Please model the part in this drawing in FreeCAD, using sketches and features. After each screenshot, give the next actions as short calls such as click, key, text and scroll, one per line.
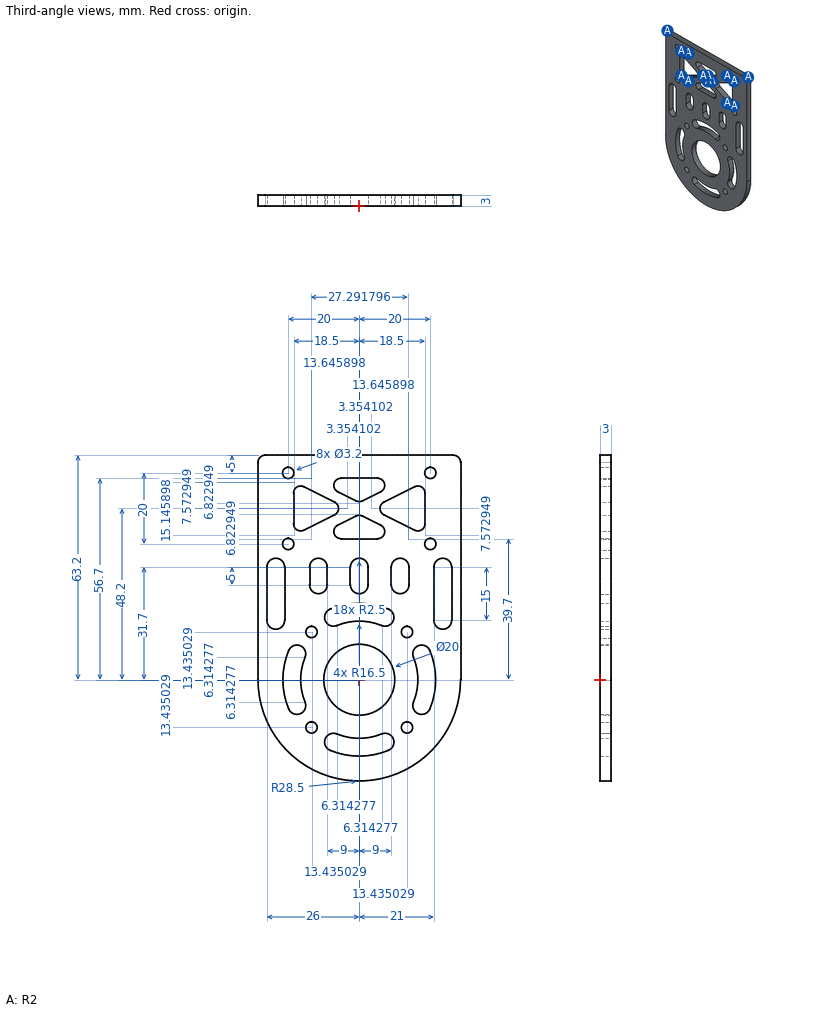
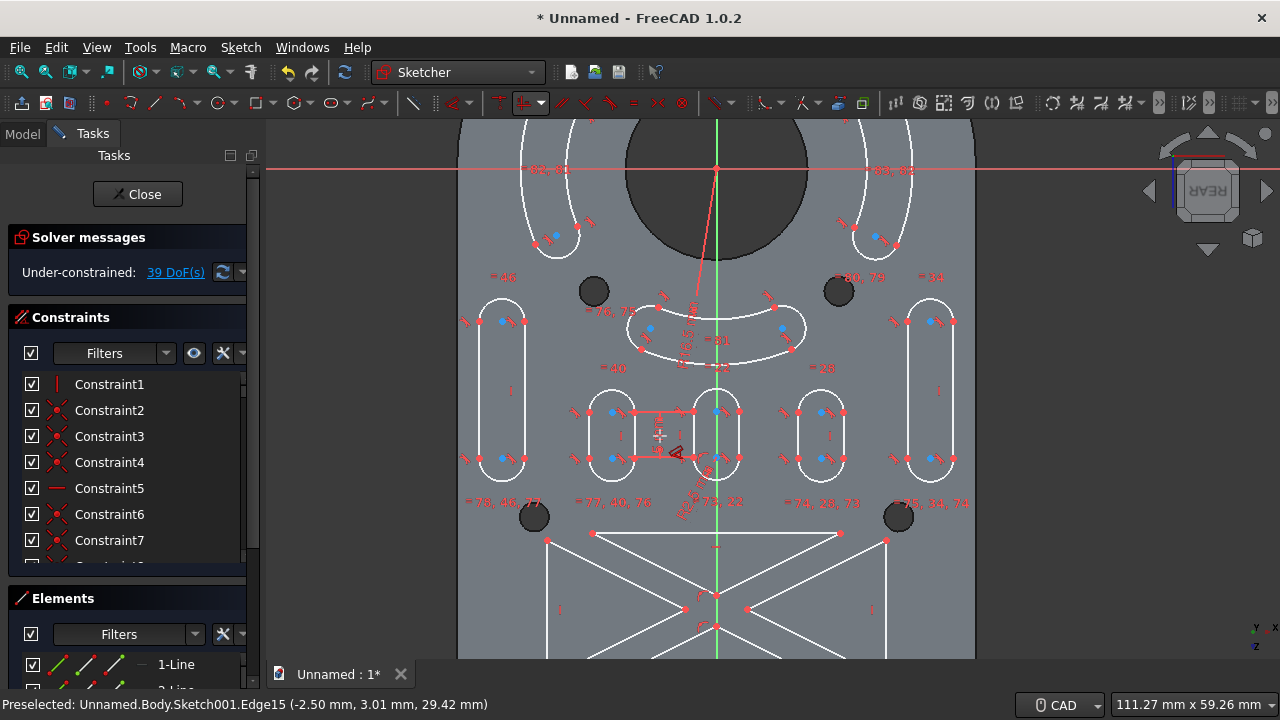
click(798, 445)
click(764, 436)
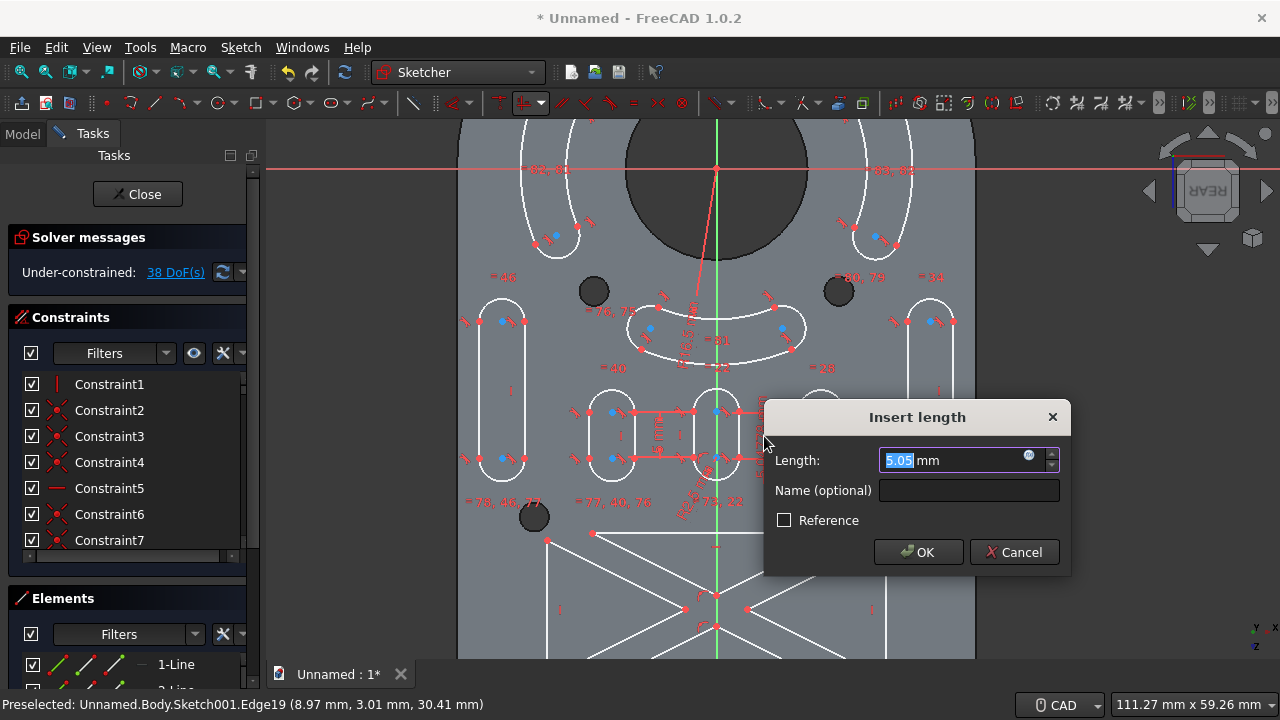
text(5)
key(Return)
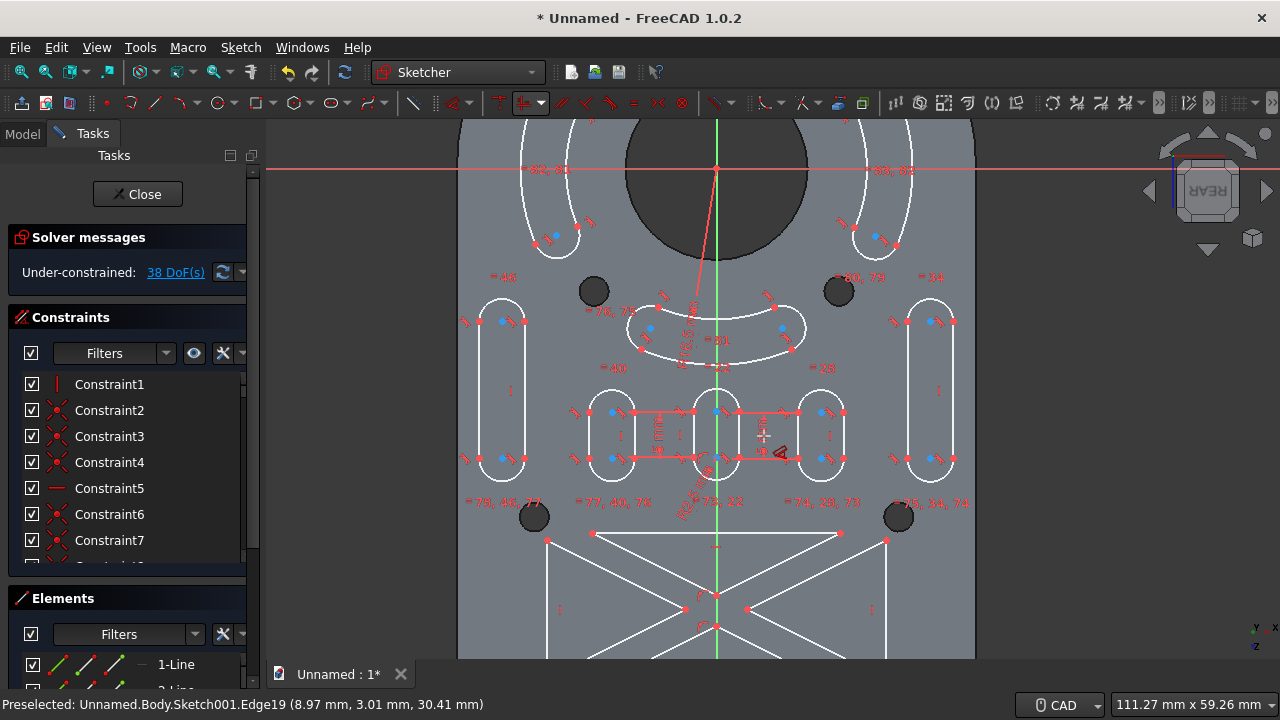
click(589, 445)
click(555, 436)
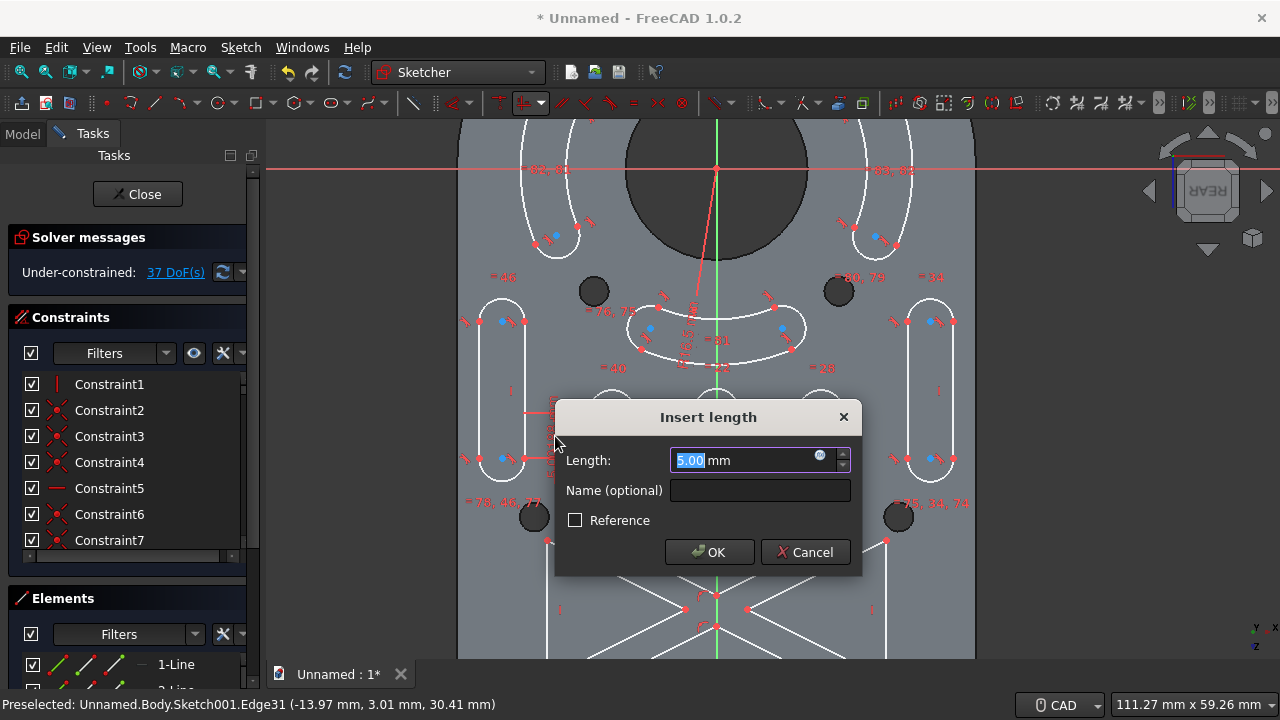
text(5)
key(Return)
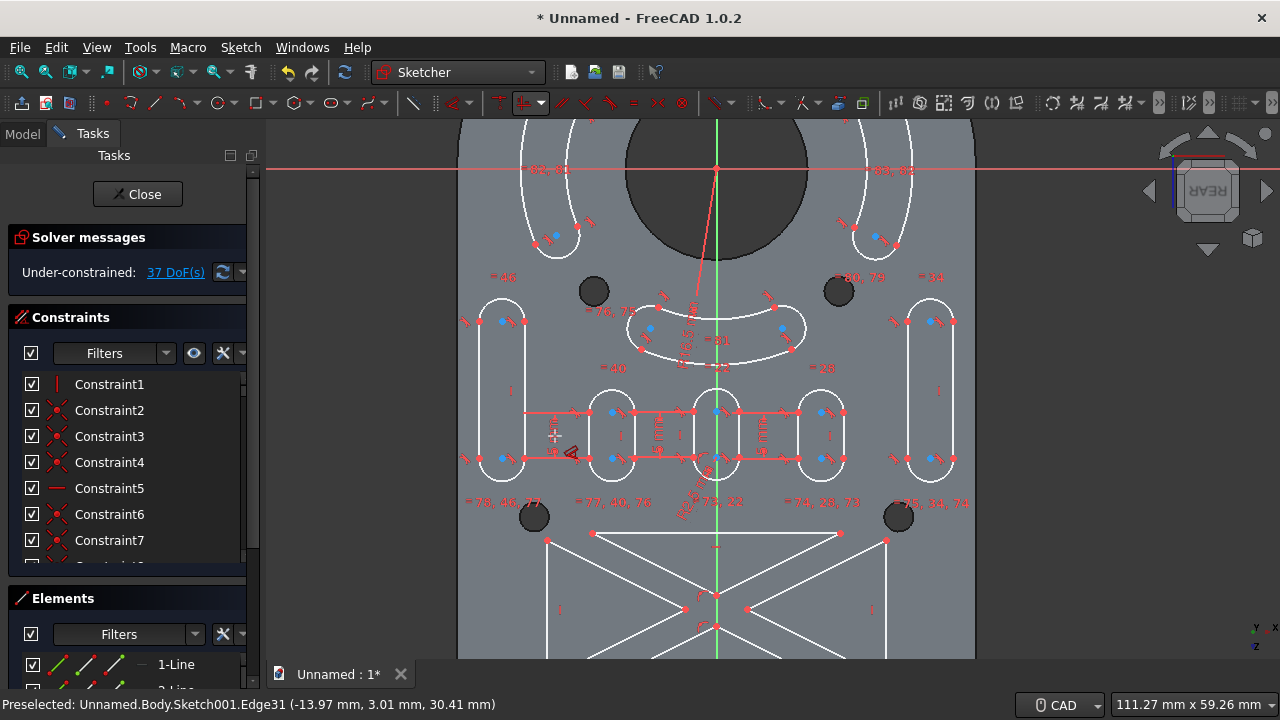
click(908, 418)
click(874, 390)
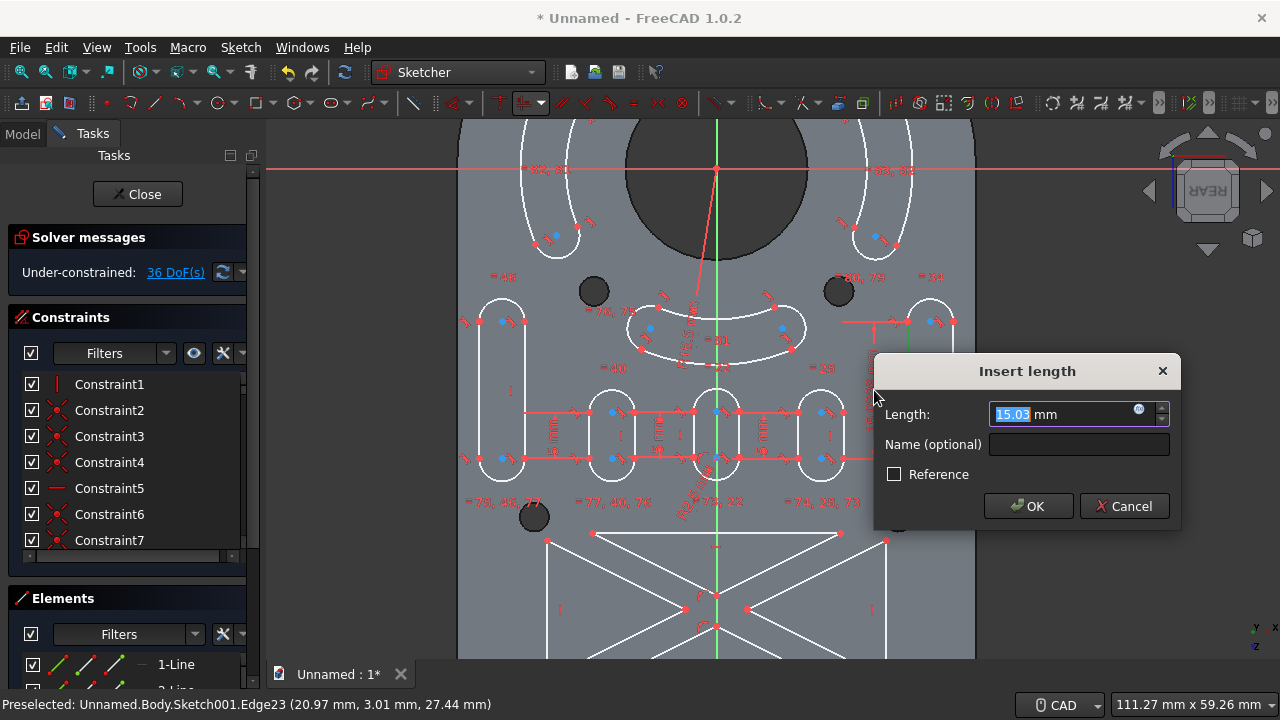
text(15)
key(Return)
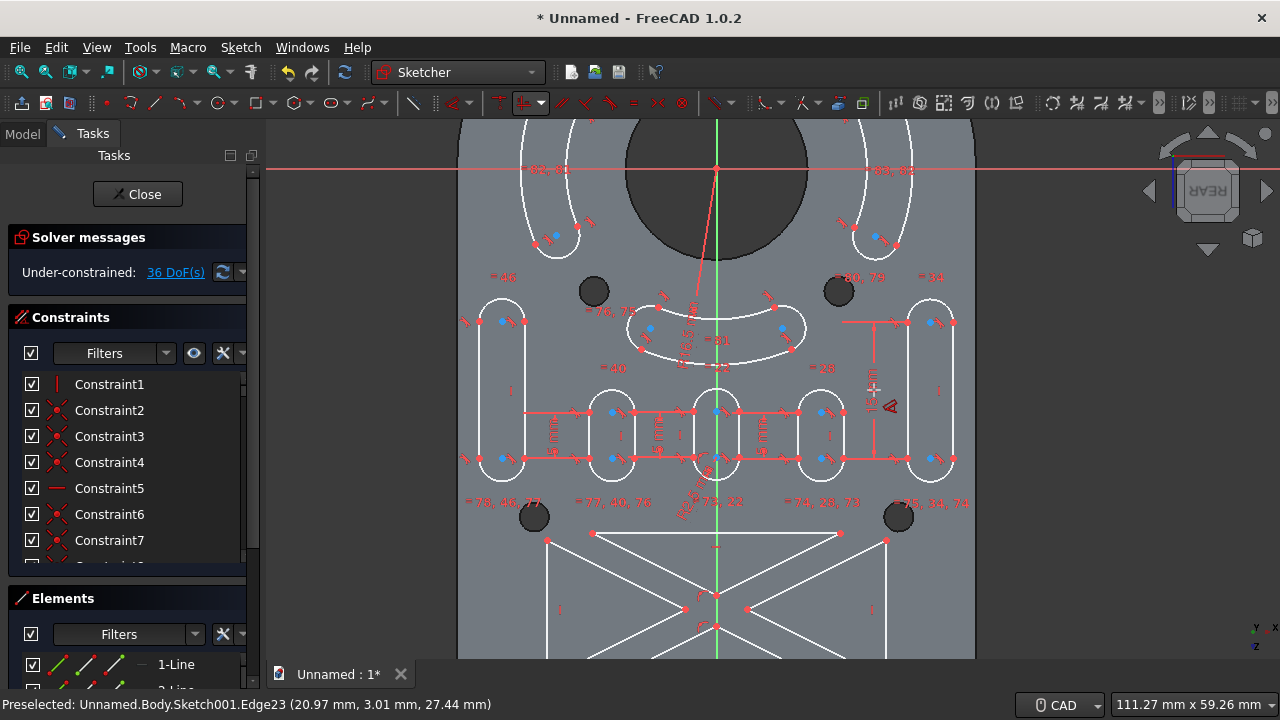
click(479, 417)
click(445, 390)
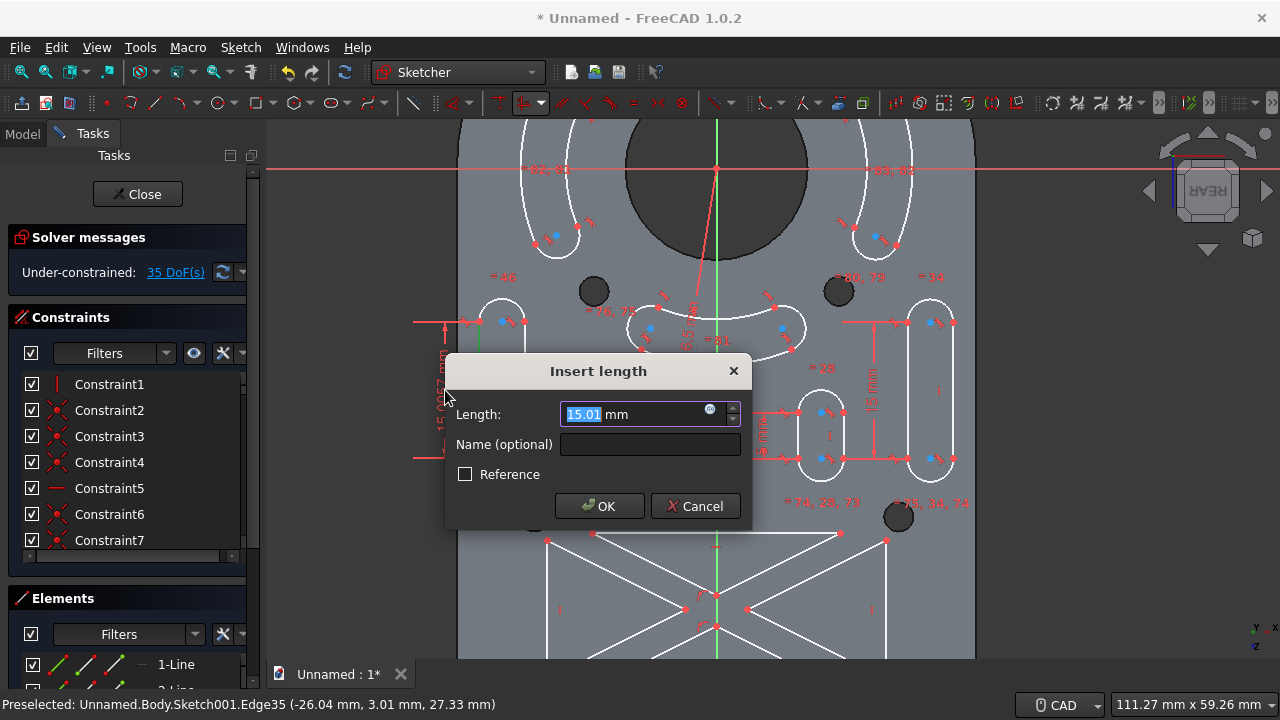
text(15)
key(Return)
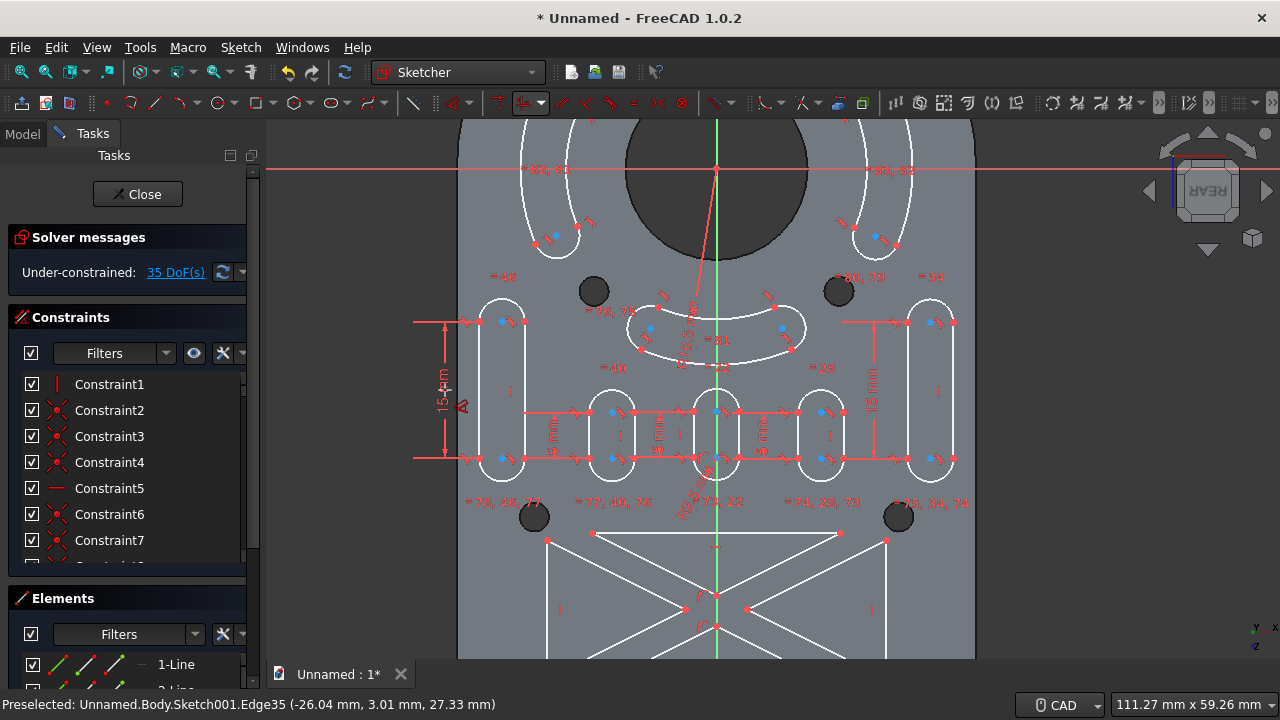
click(798, 459)
click(776, 493)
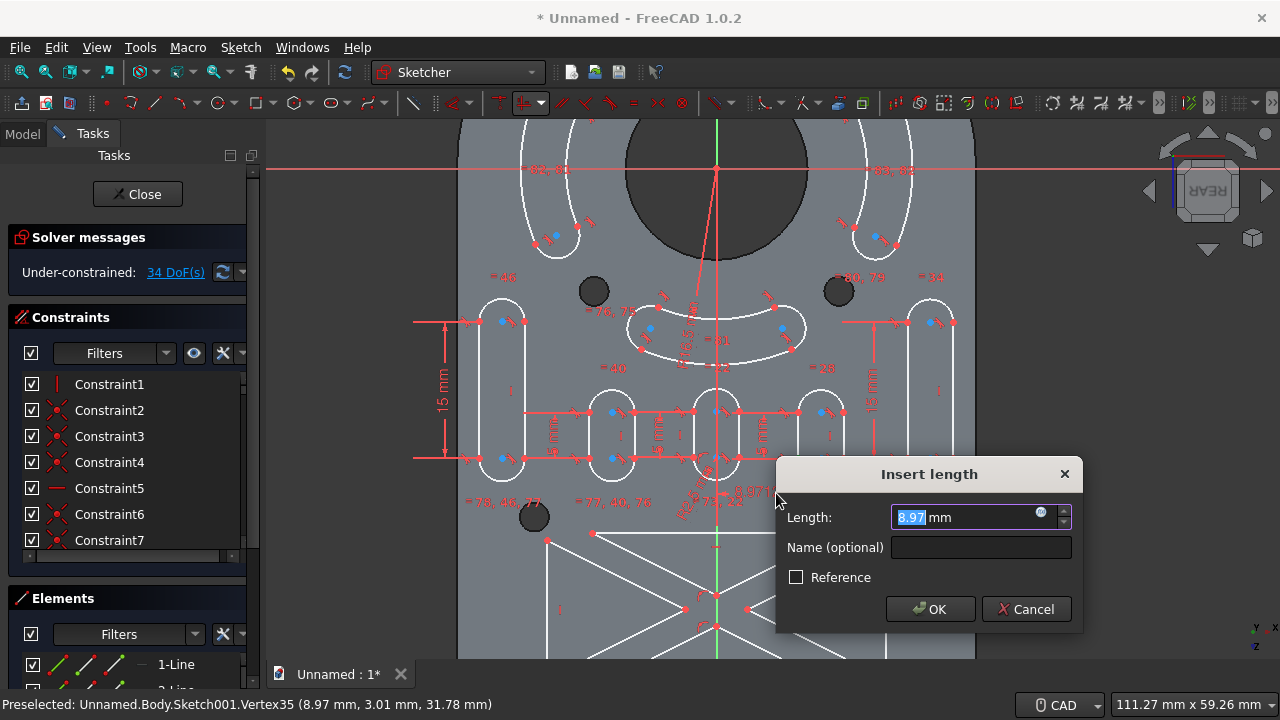
text(9)
key(Return)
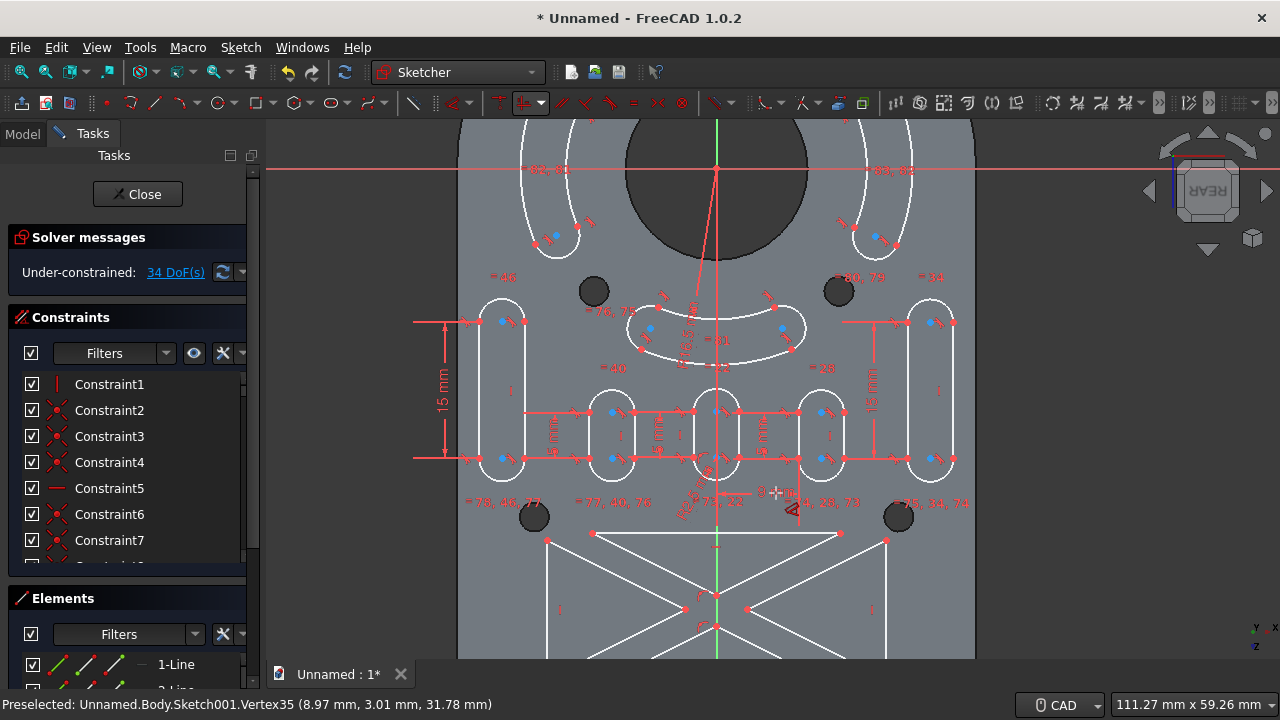
click(635, 458)
click(676, 516)